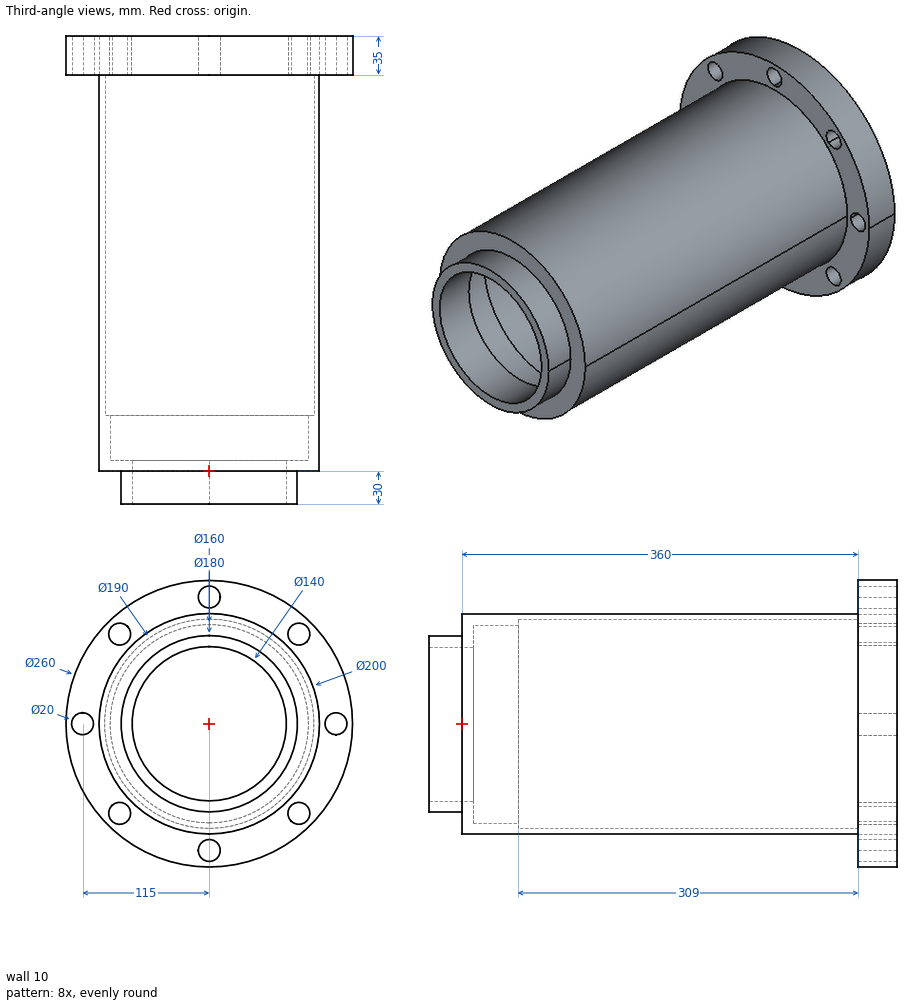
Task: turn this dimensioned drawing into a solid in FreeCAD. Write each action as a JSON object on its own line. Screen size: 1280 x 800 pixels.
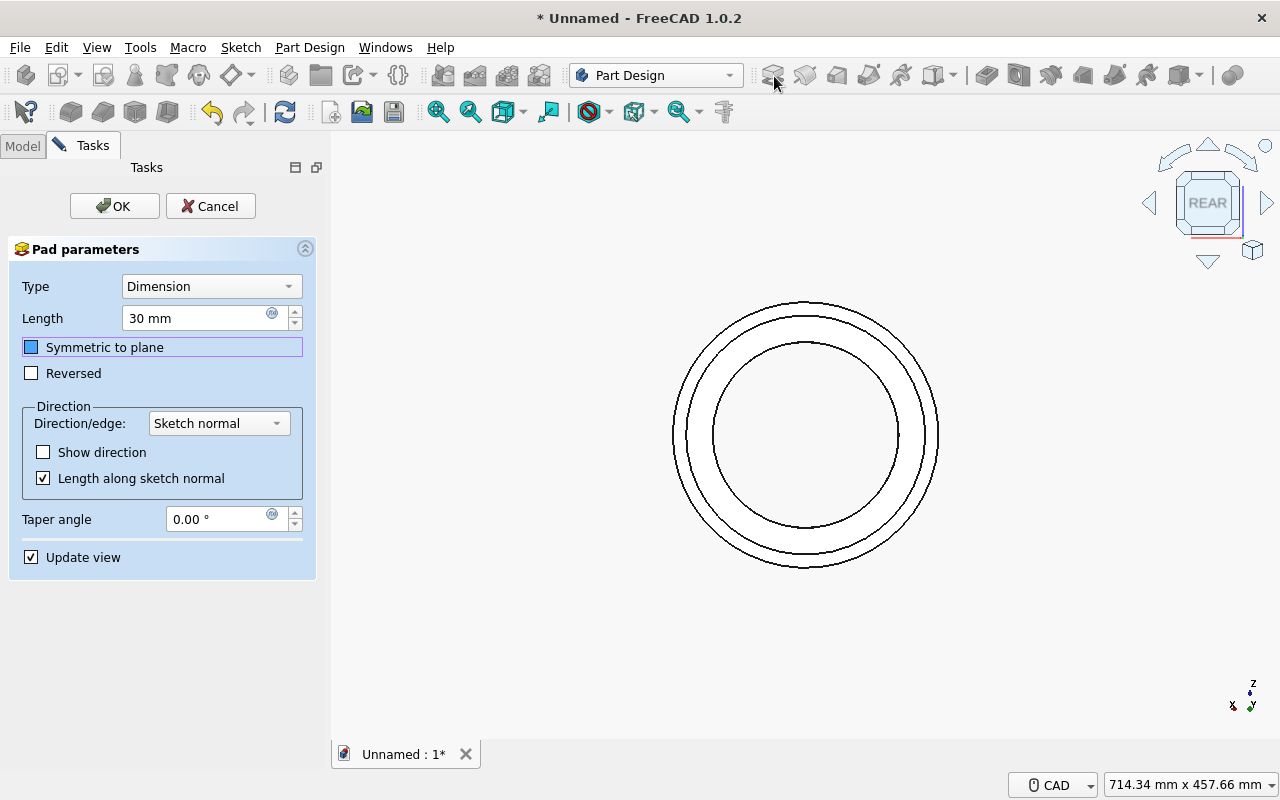
{"action": "left_click", "coordinate": [115, 206]}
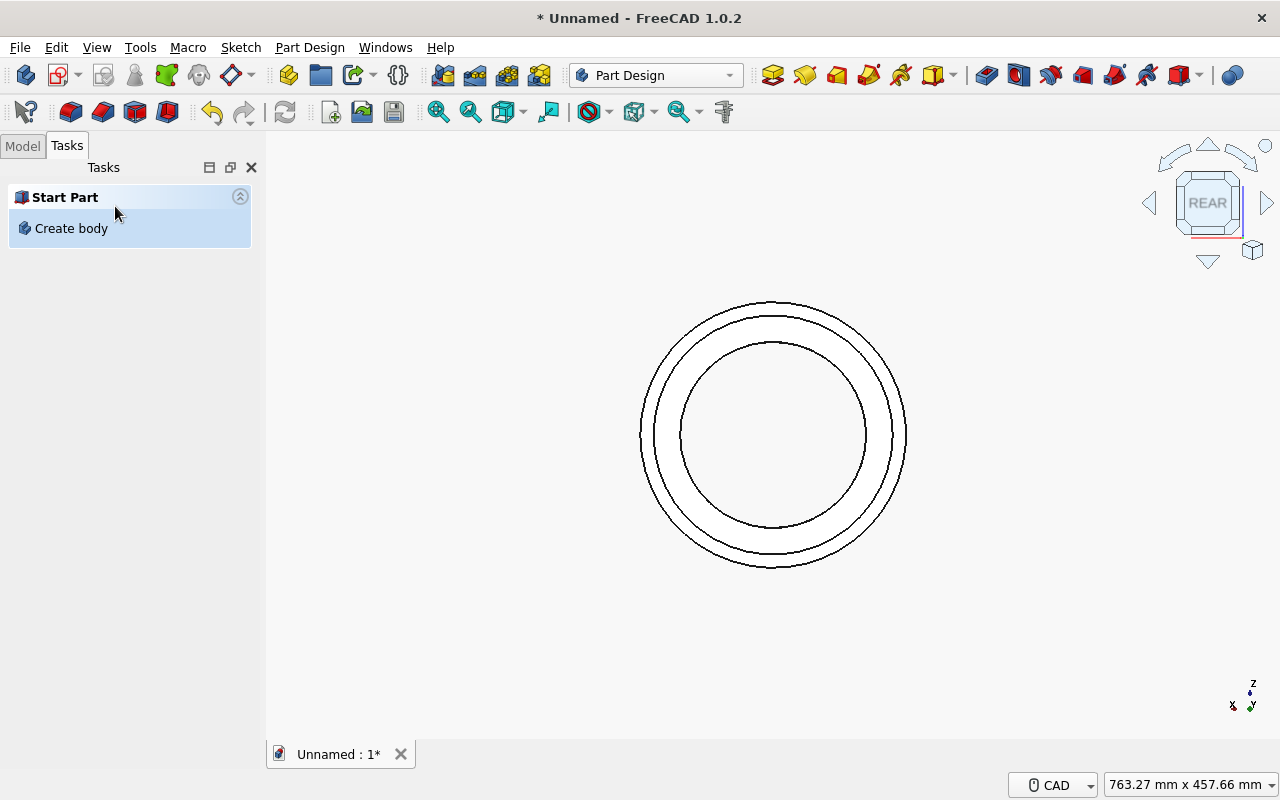
{"action": "left_click", "coordinate": [440, 112]}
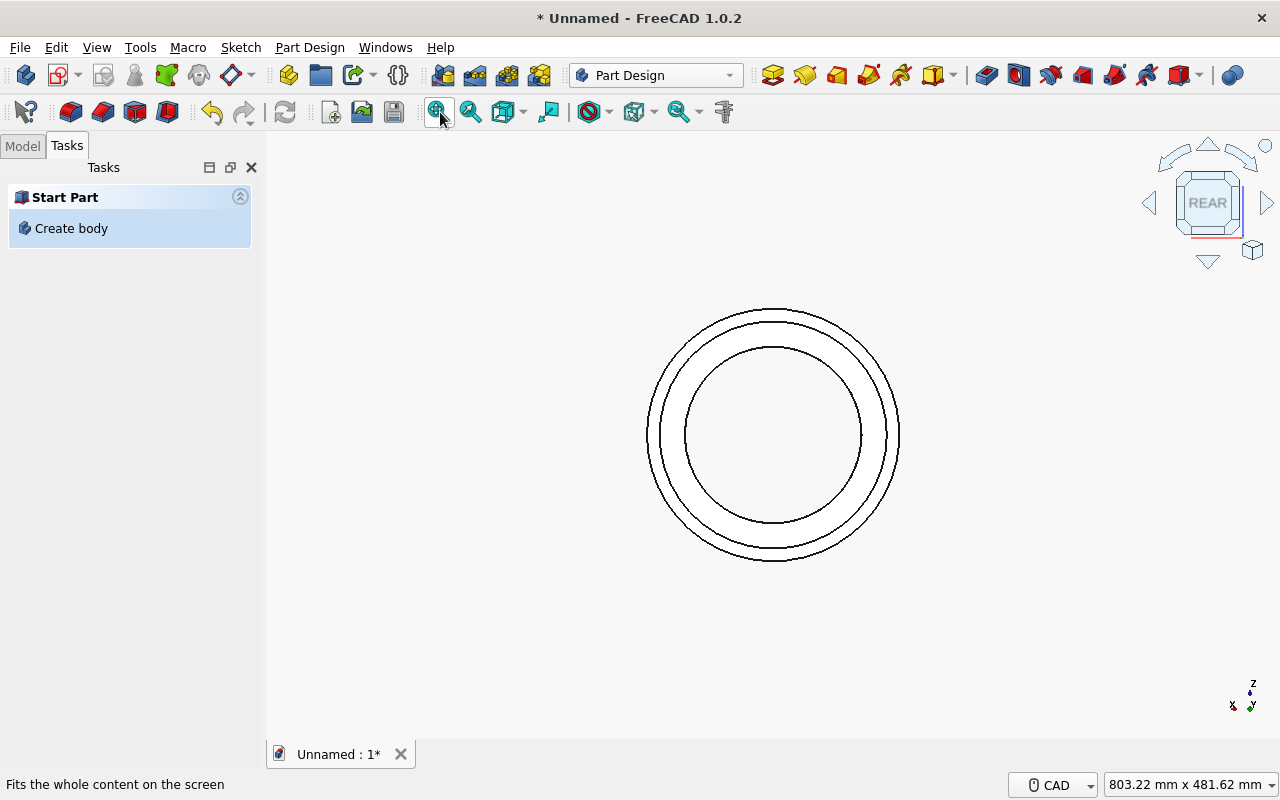
{"action": "scroll", "coordinate": [737, 326], "scroll_direction": "up", "scroll_amount": 15}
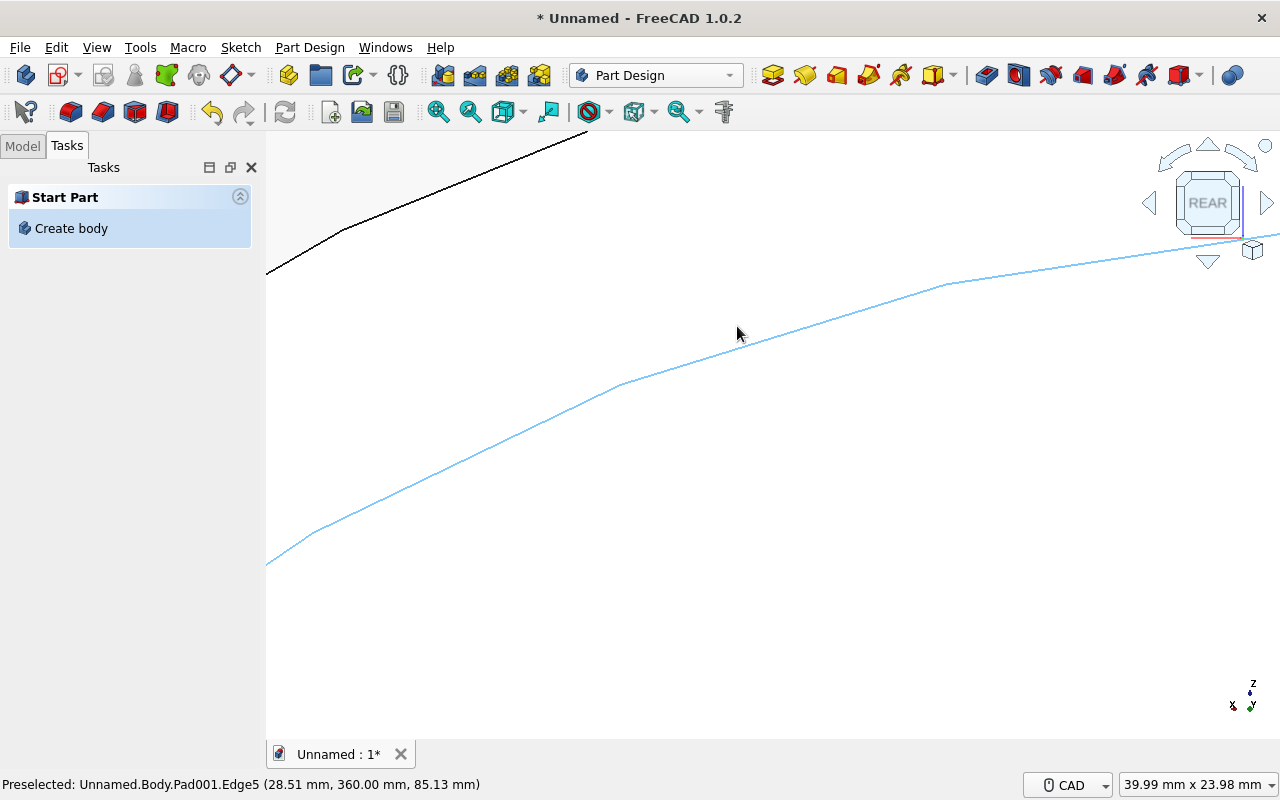
{"action": "left_click", "coordinate": [730, 335]}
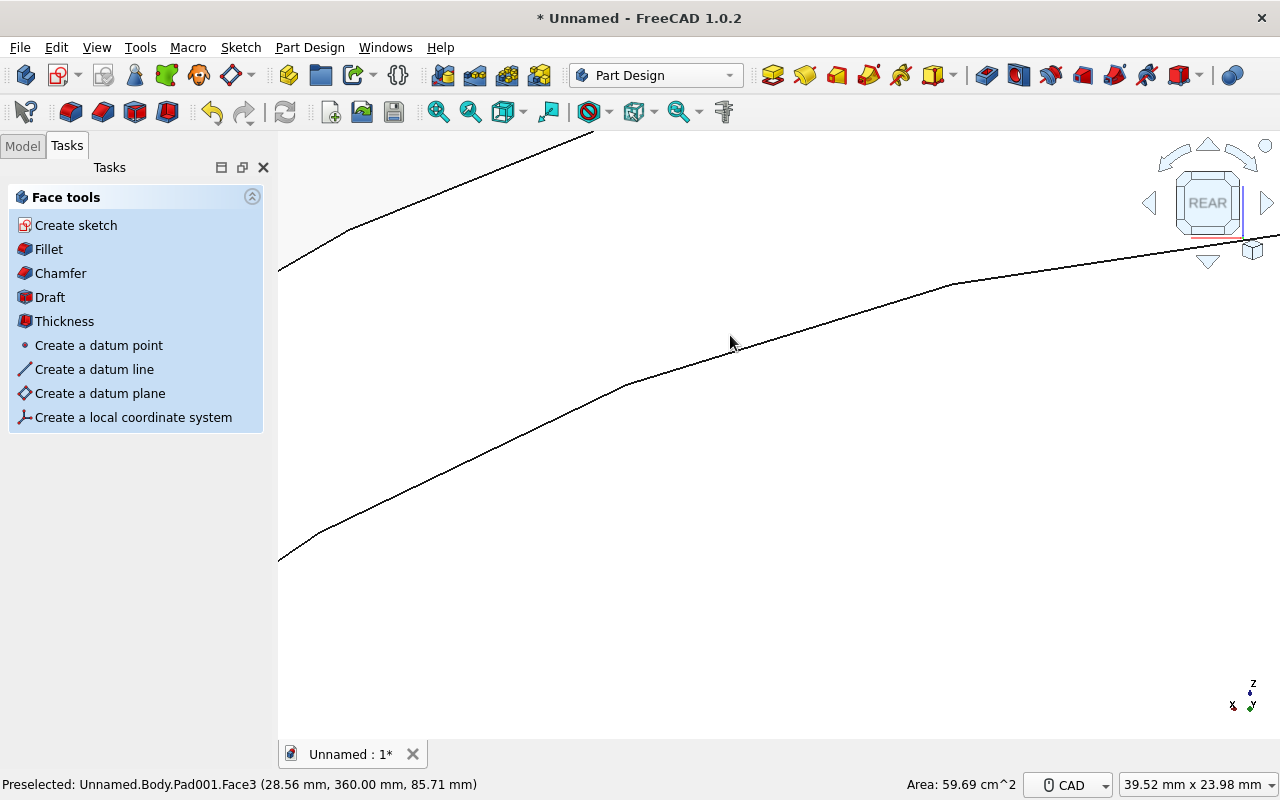
{"action": "left_click", "coordinate": [58, 76]}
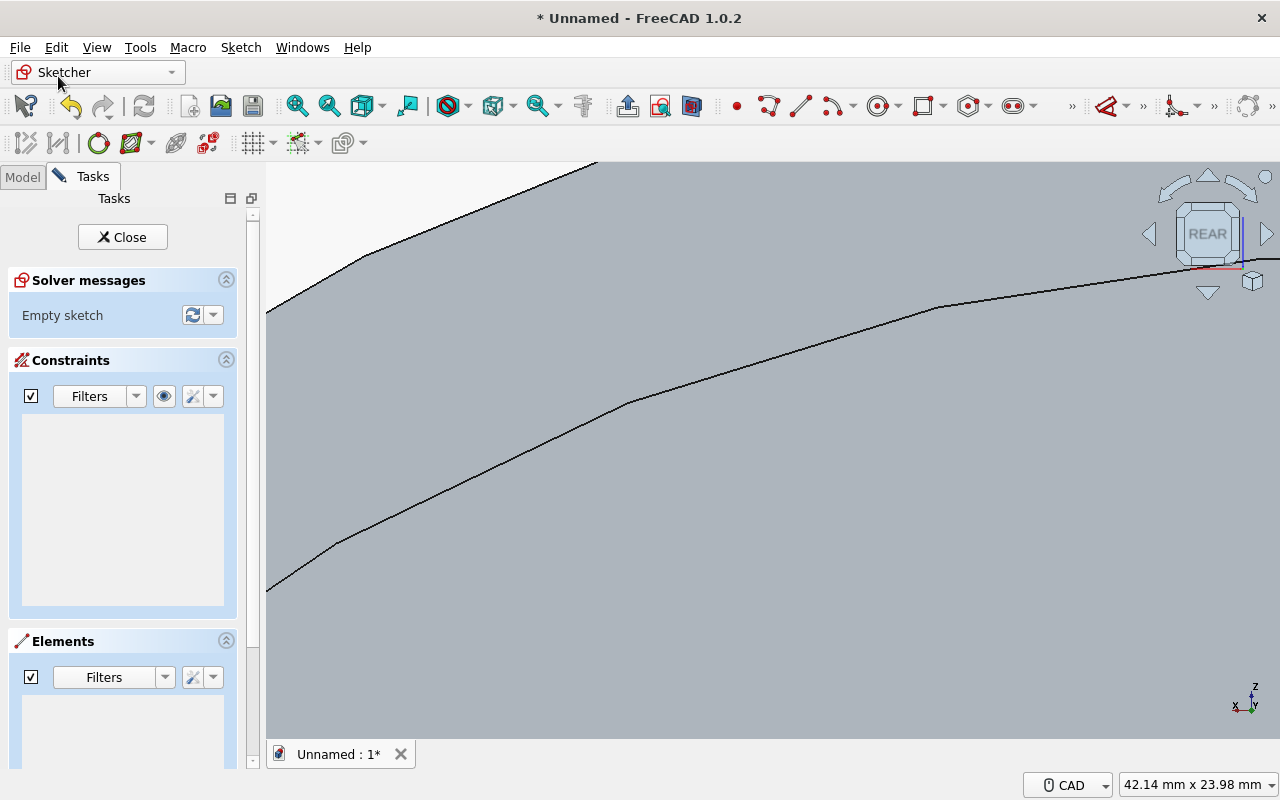
{"action": "scroll", "coordinate": [647, 293], "scroll_direction": "down", "scroll_amount": 13}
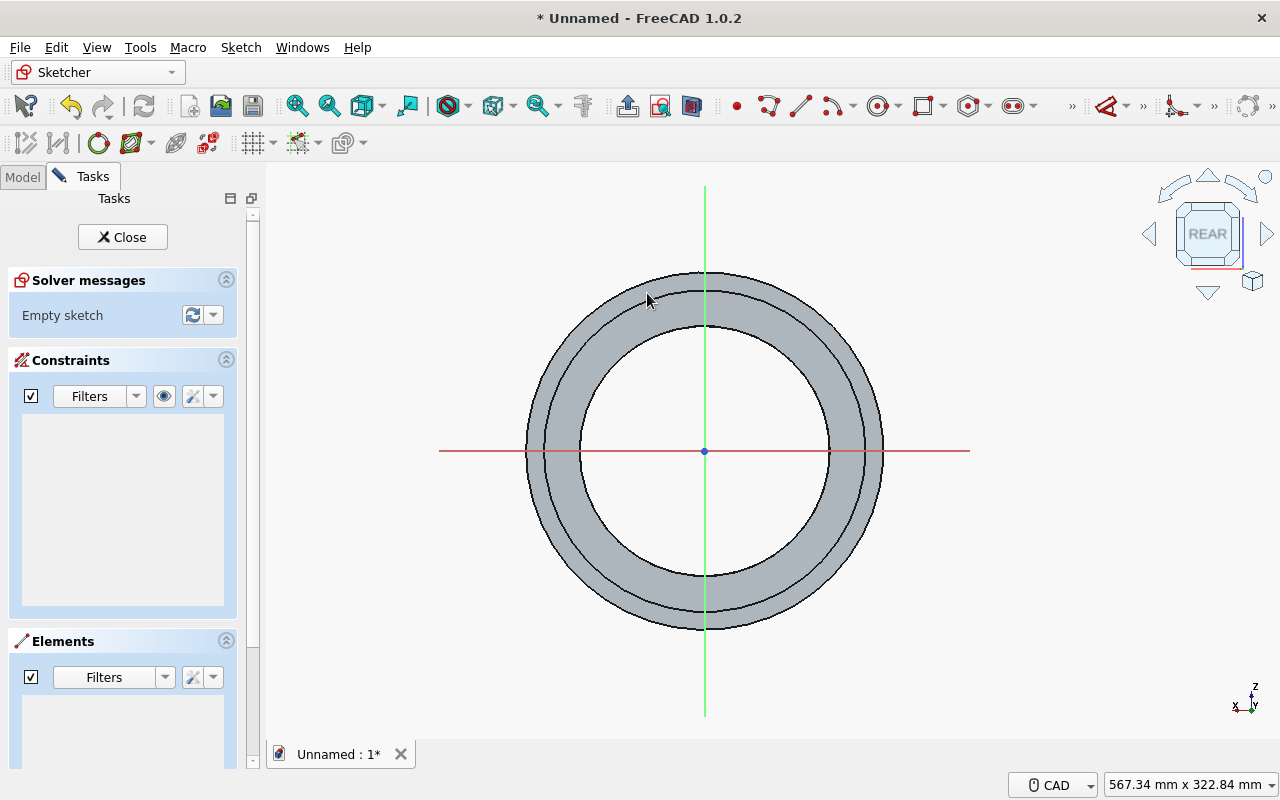
{"action": "left_click", "coordinate": [878, 106]}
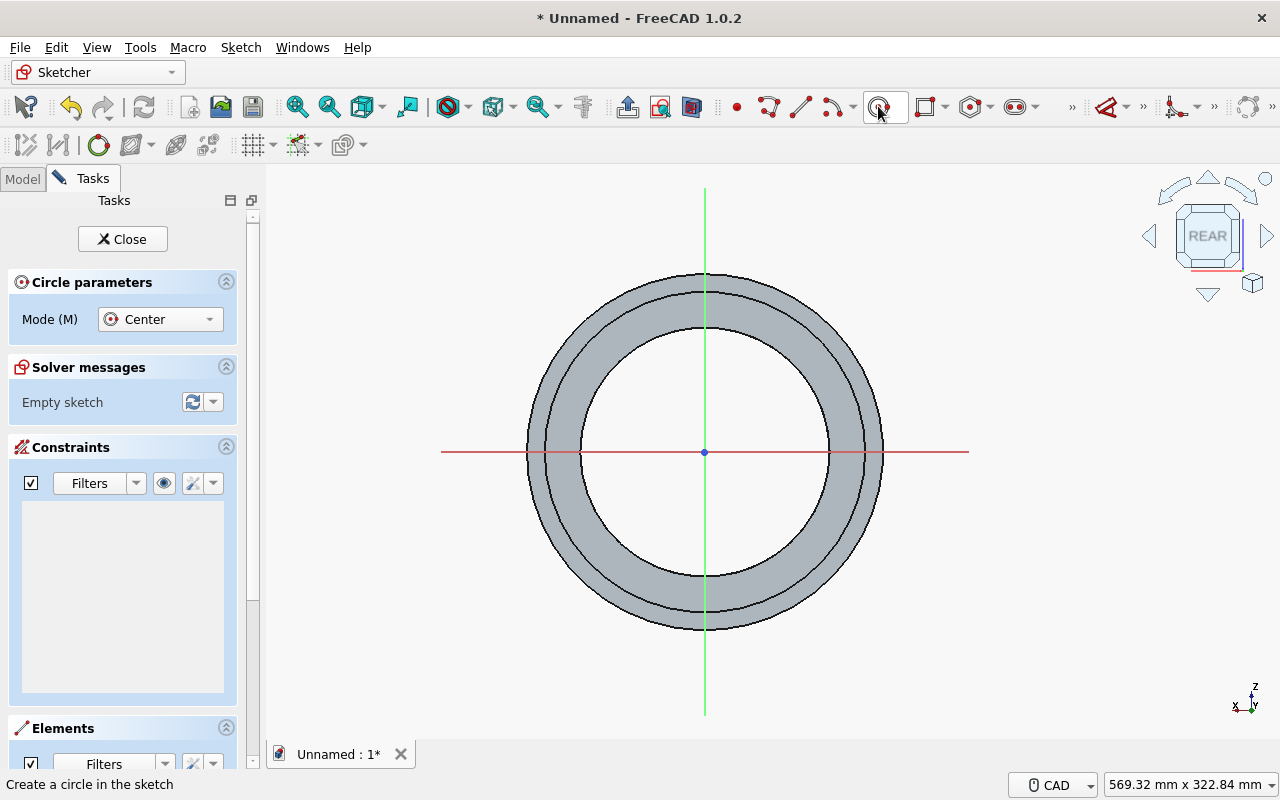
{"action": "left_click", "coordinate": [705, 452]}
{"action": "left_click", "coordinate": [825, 332]}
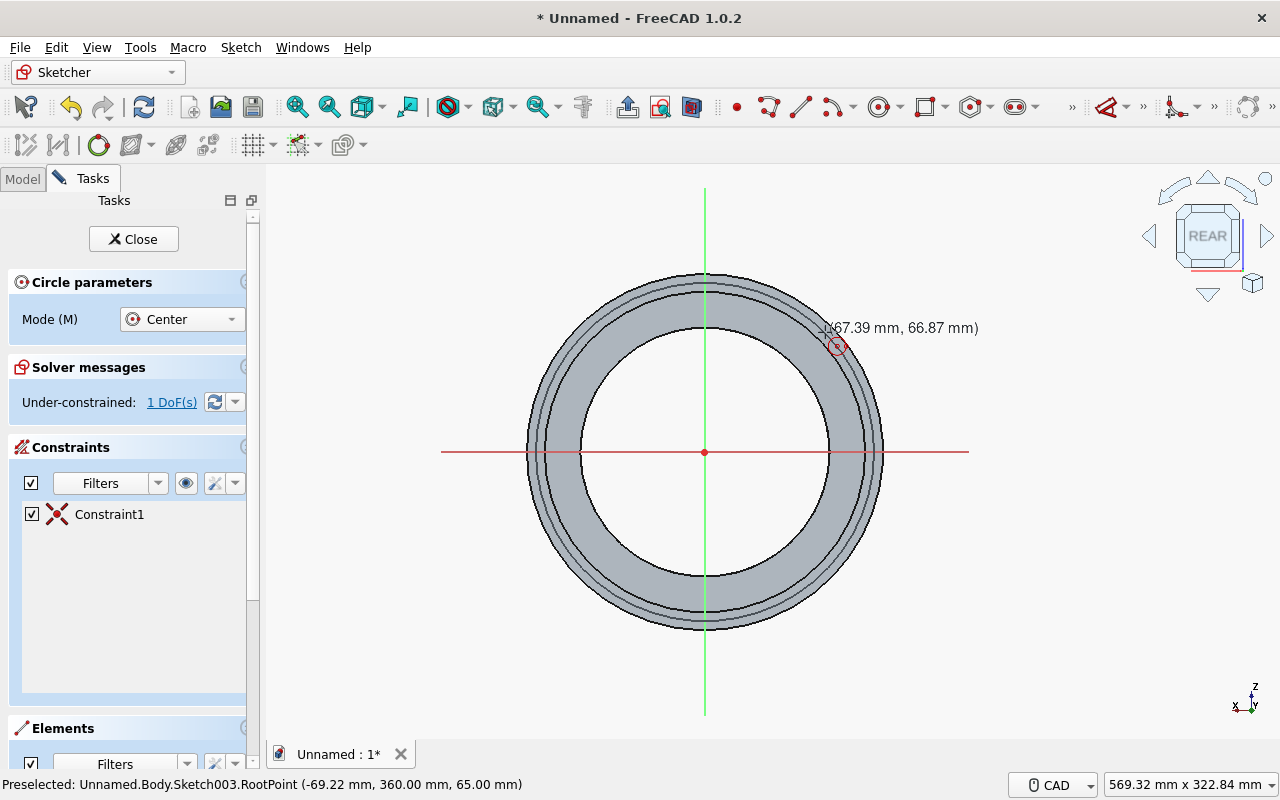
{"action": "left_click", "coordinate": [705, 452]}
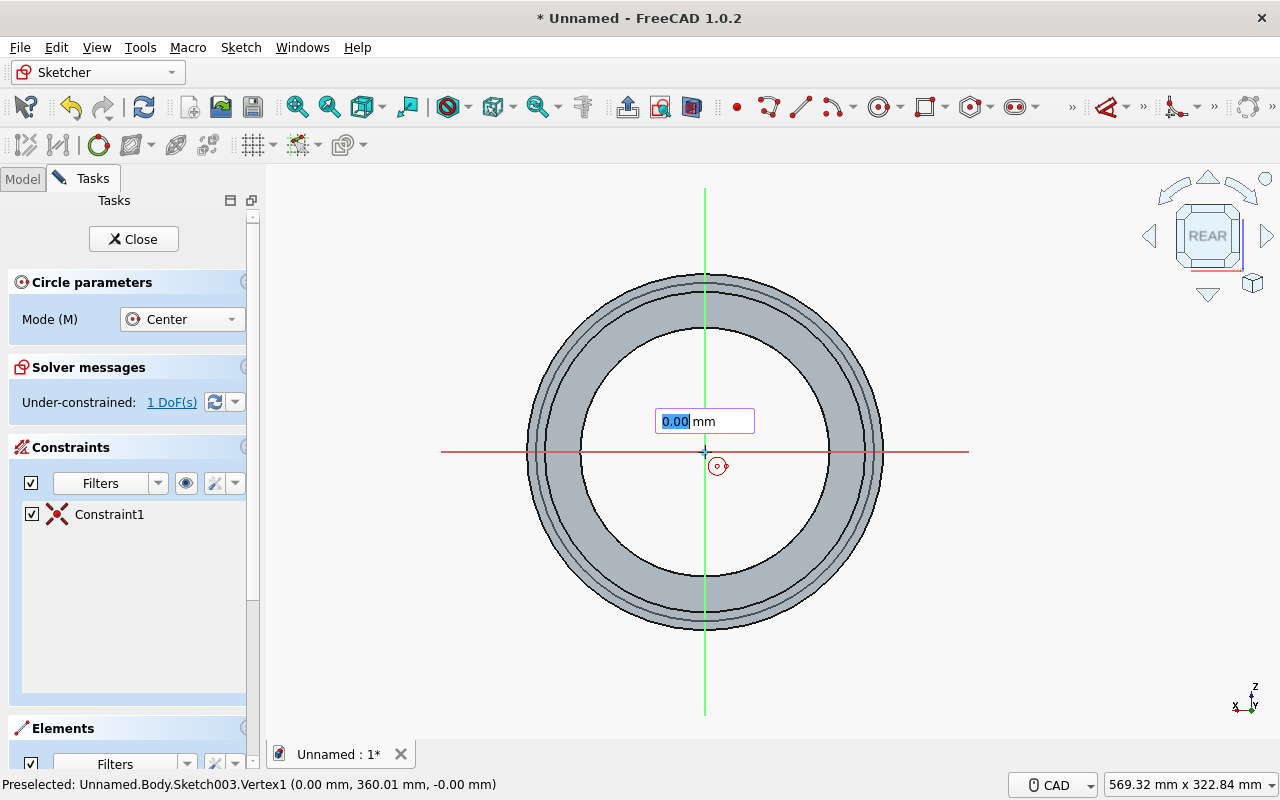
{"action": "scroll", "coordinate": [818, 339], "scroll_direction": "up", "scroll_amount": 3}